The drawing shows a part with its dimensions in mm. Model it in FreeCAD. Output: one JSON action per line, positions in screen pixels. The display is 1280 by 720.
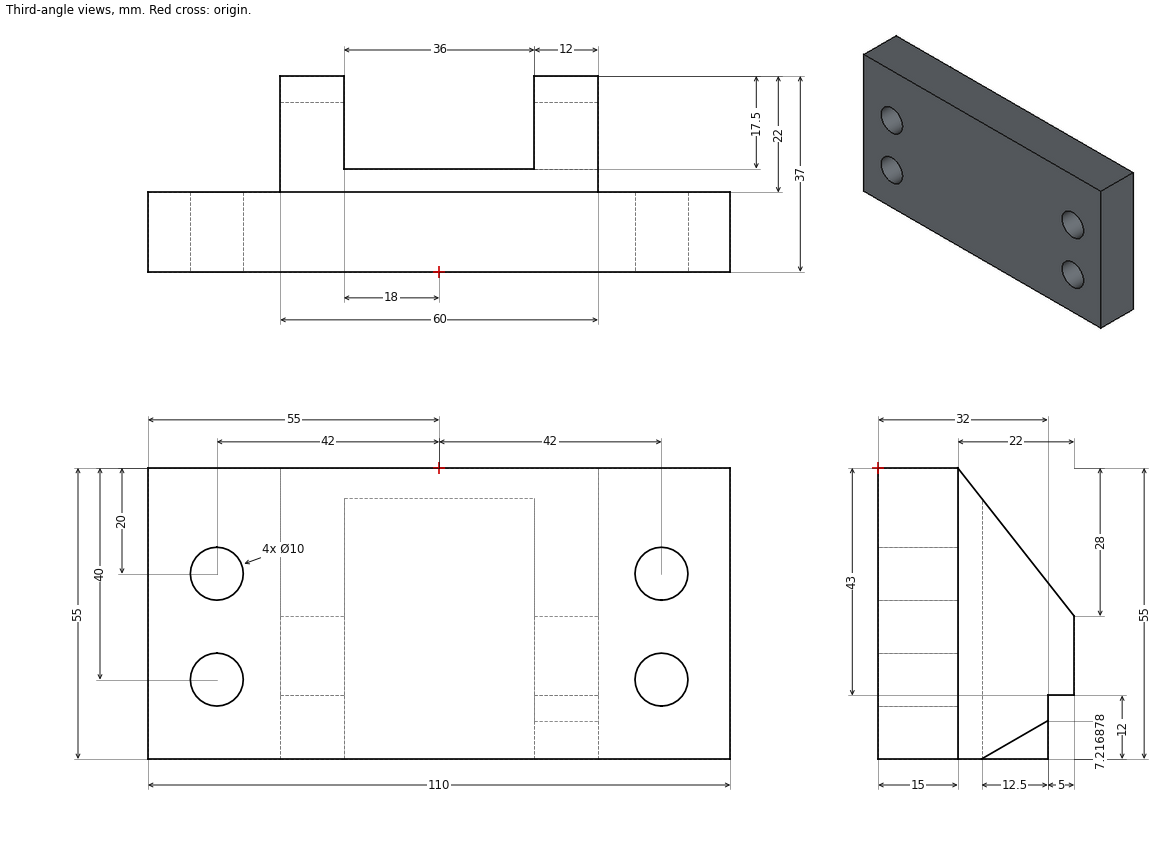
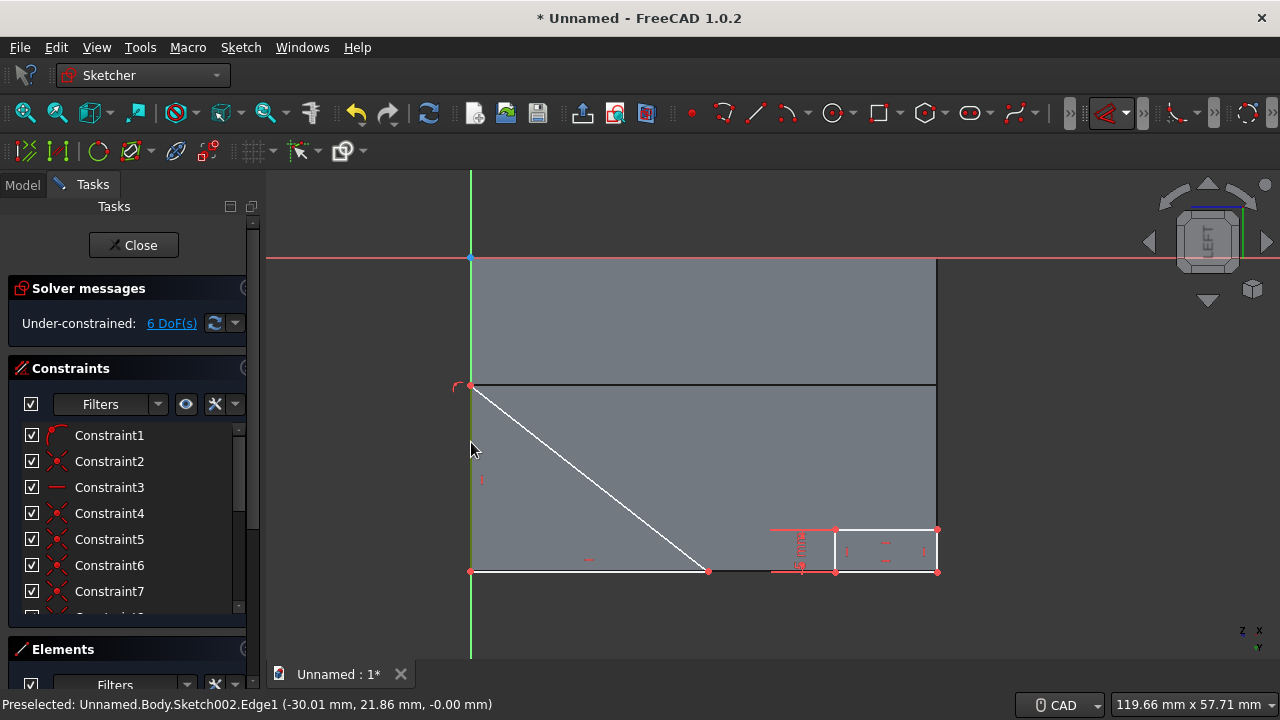
{"action": "left_click", "coordinate": [1128, 114]}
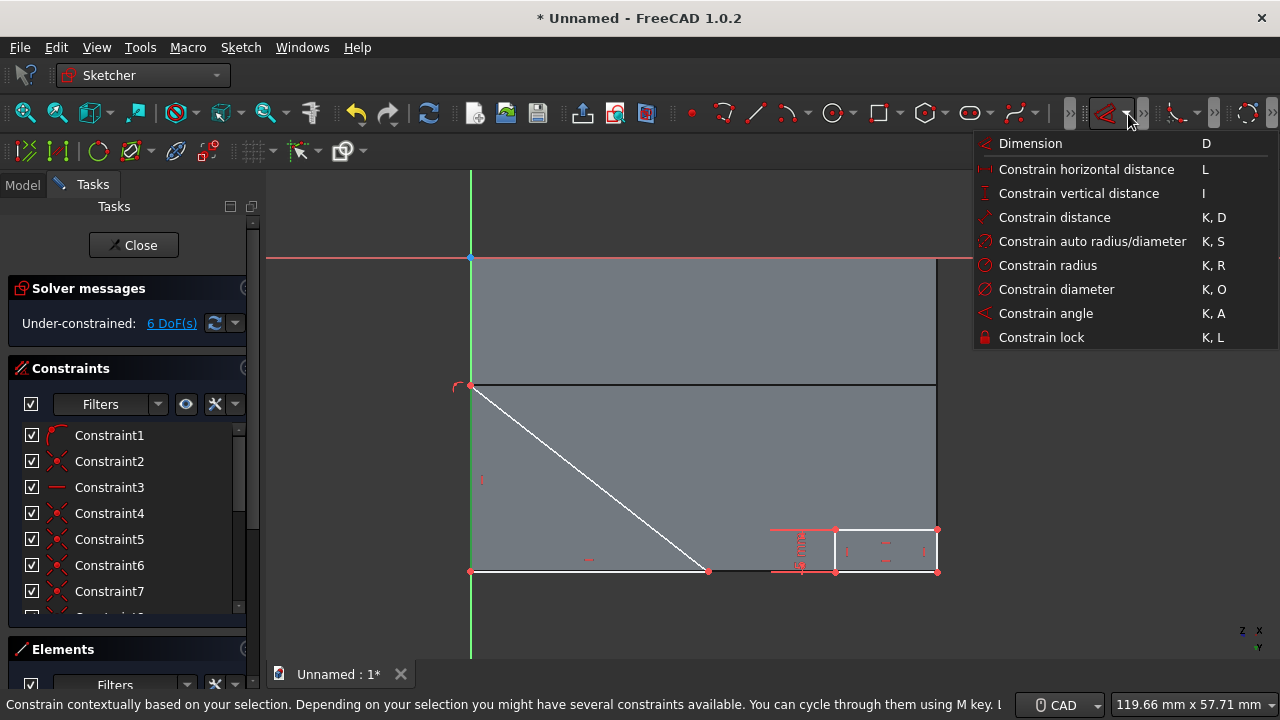
{"action": "left_click", "coordinate": [1126, 193]}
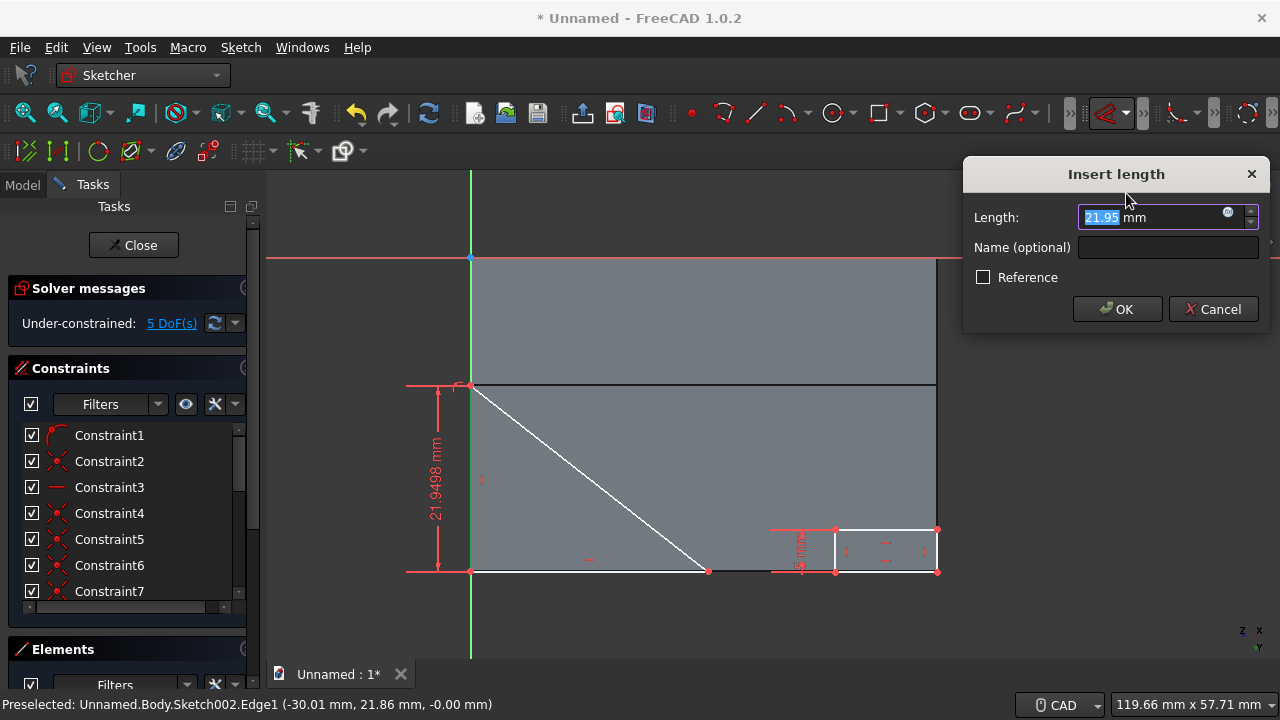
{"action": "type", "text": "22"}
{"action": "key", "text": "Return"}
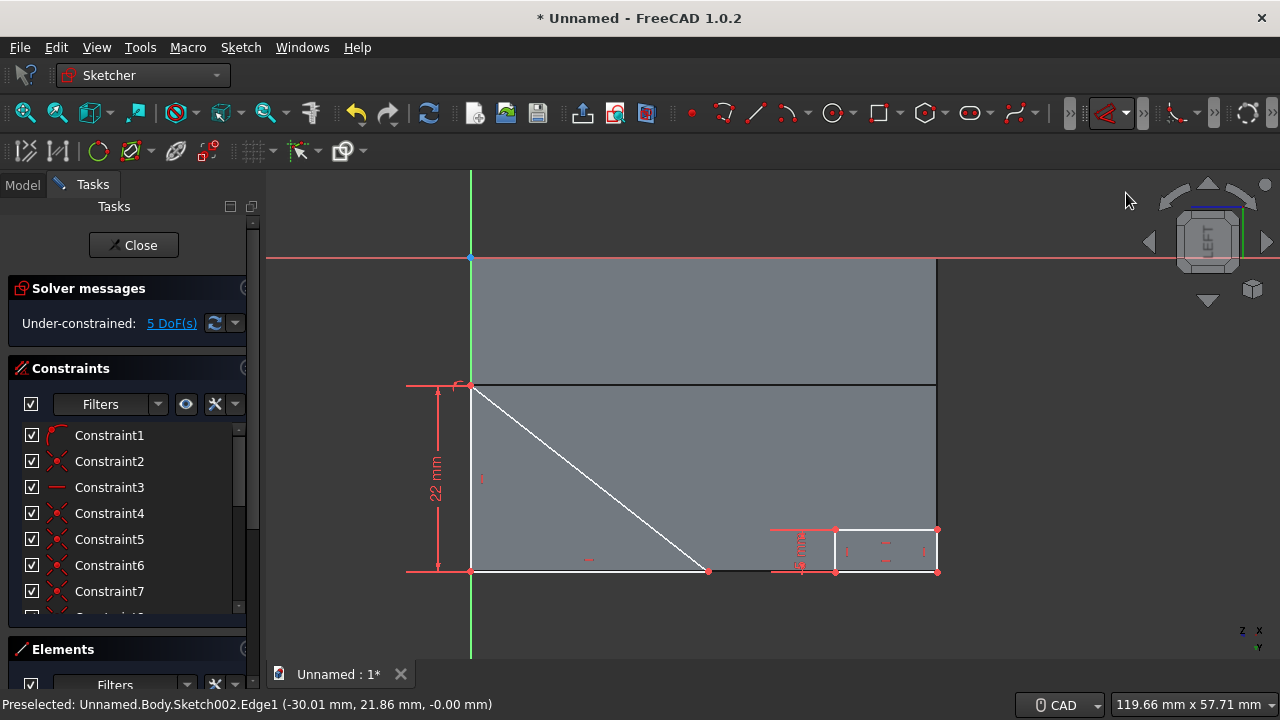
{"action": "left_click", "coordinate": [542, 572]}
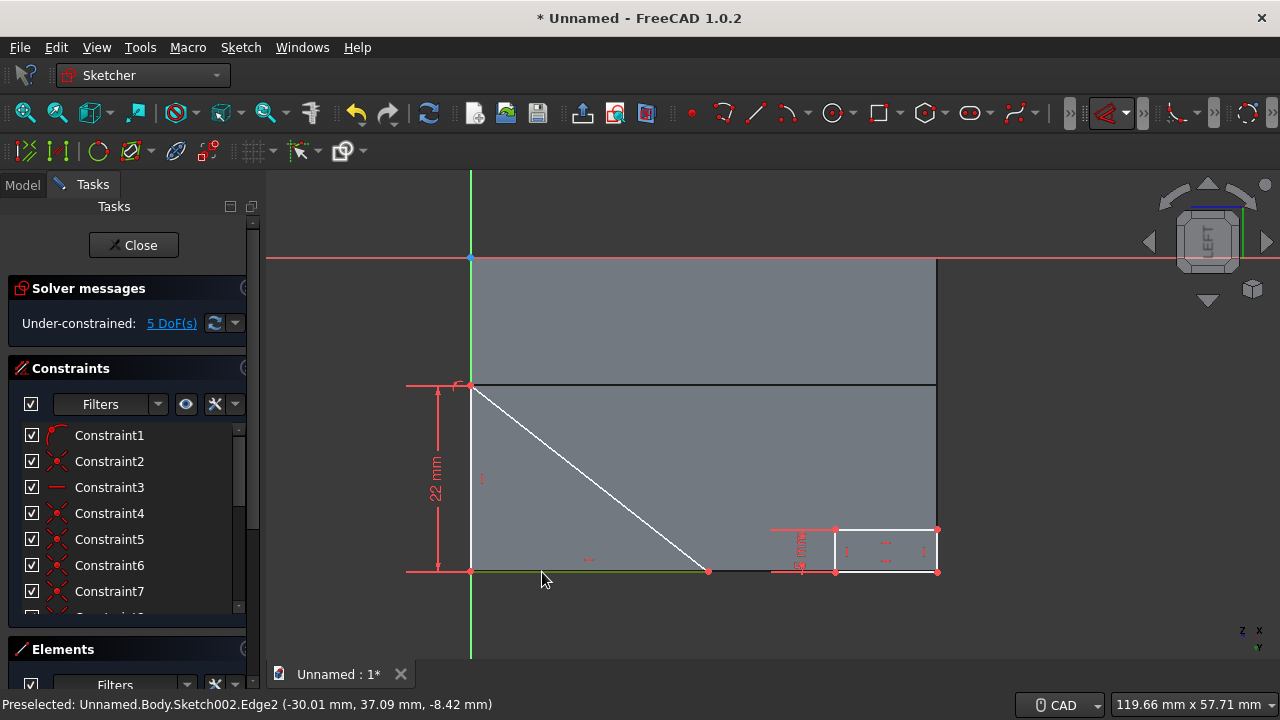
{"action": "left_click", "coordinate": [1128, 114]}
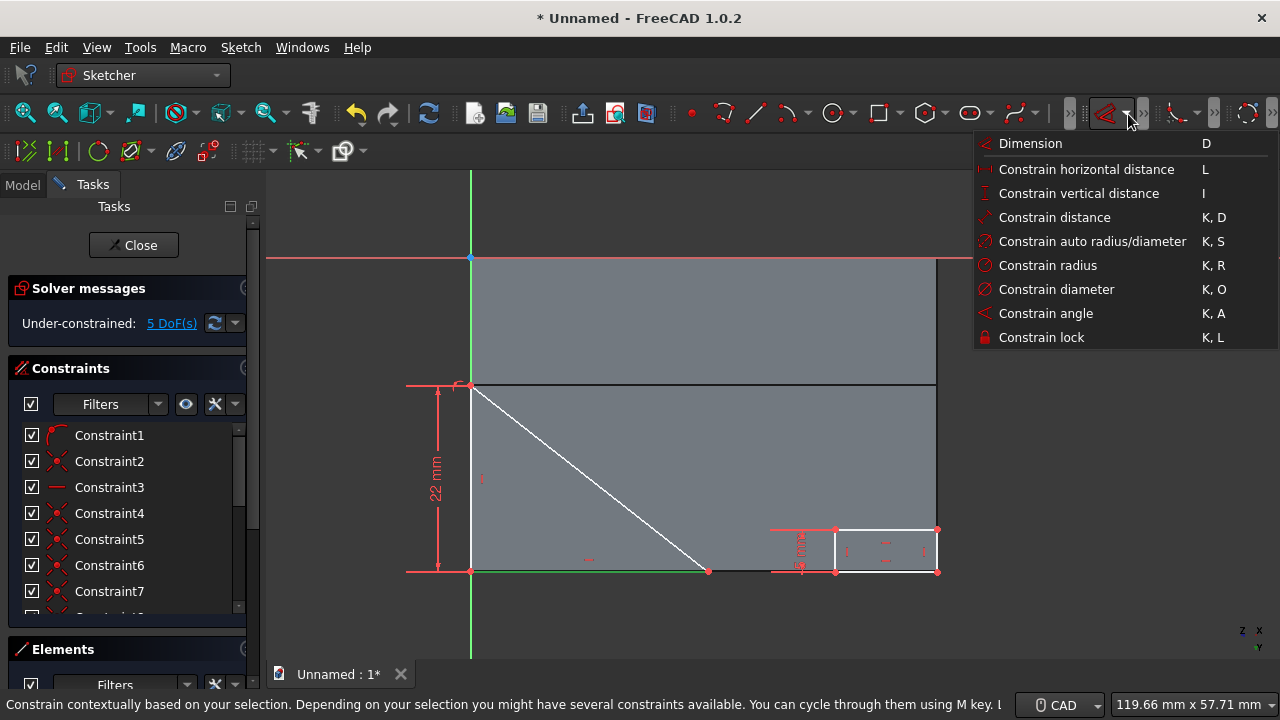
{"action": "left_click", "coordinate": [1126, 169]}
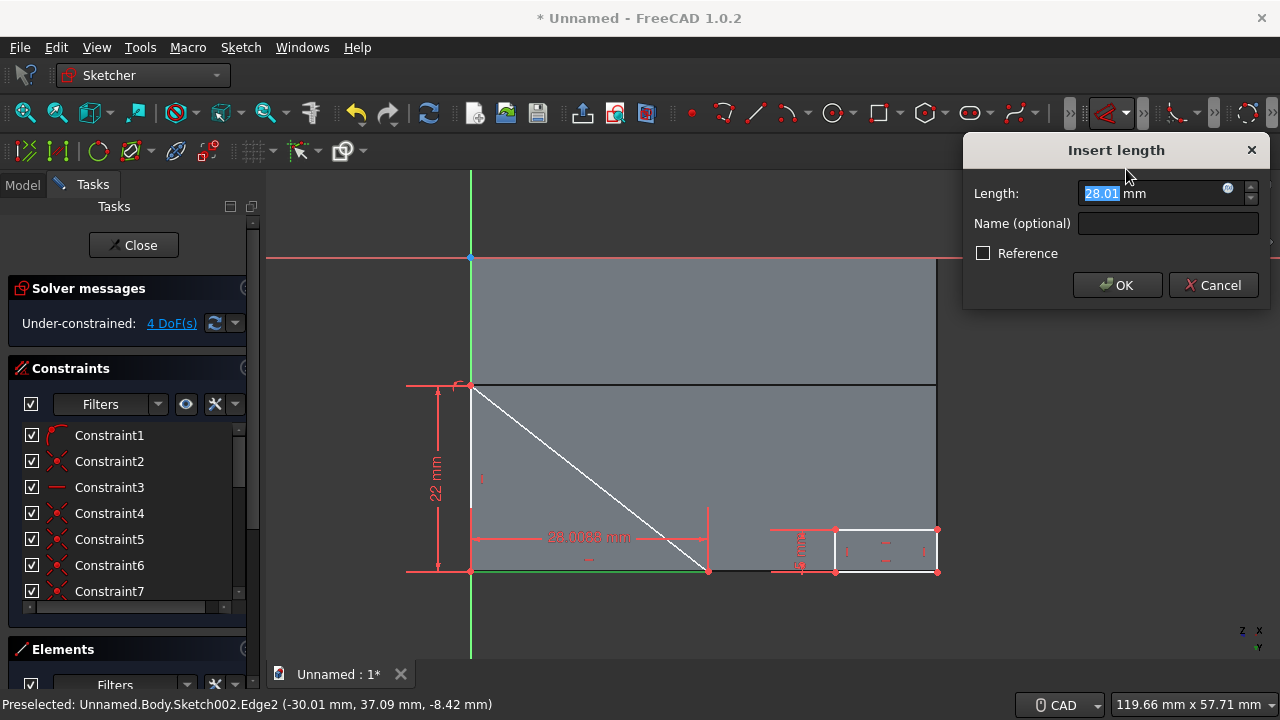
{"action": "type", "text": "28"}
{"action": "key", "text": "Return"}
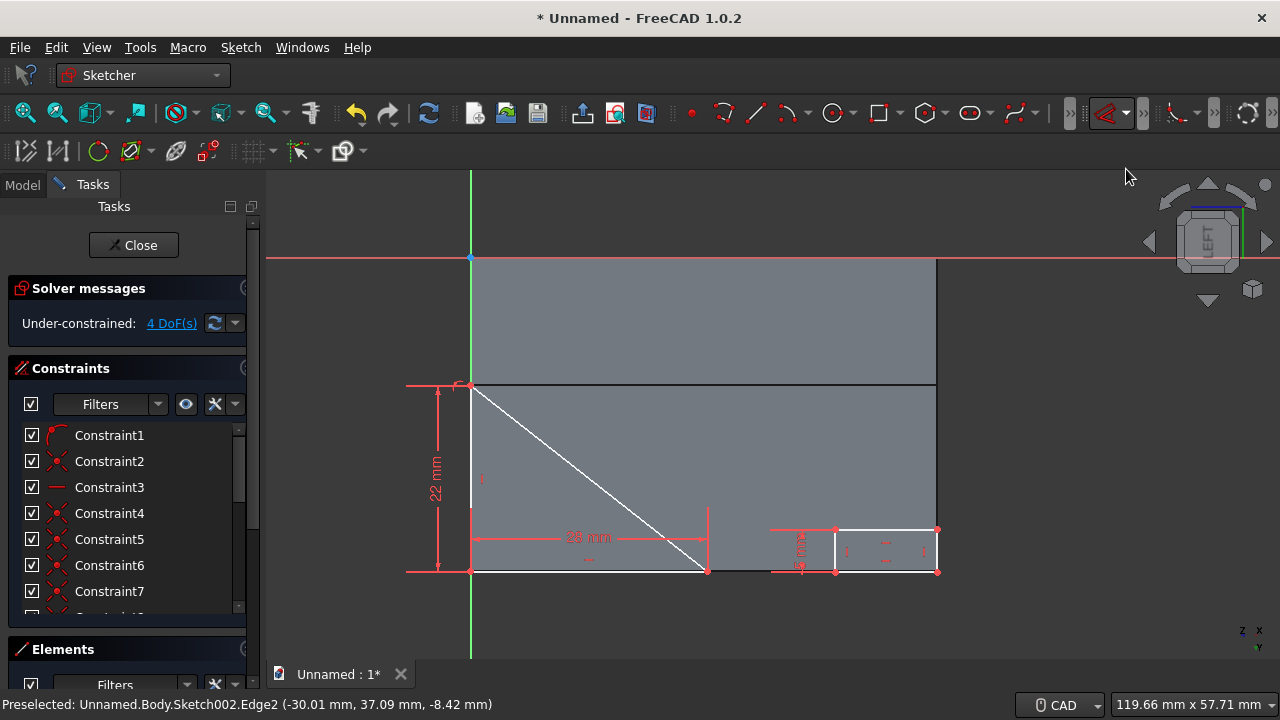
{"action": "left_click", "coordinate": [866, 572]}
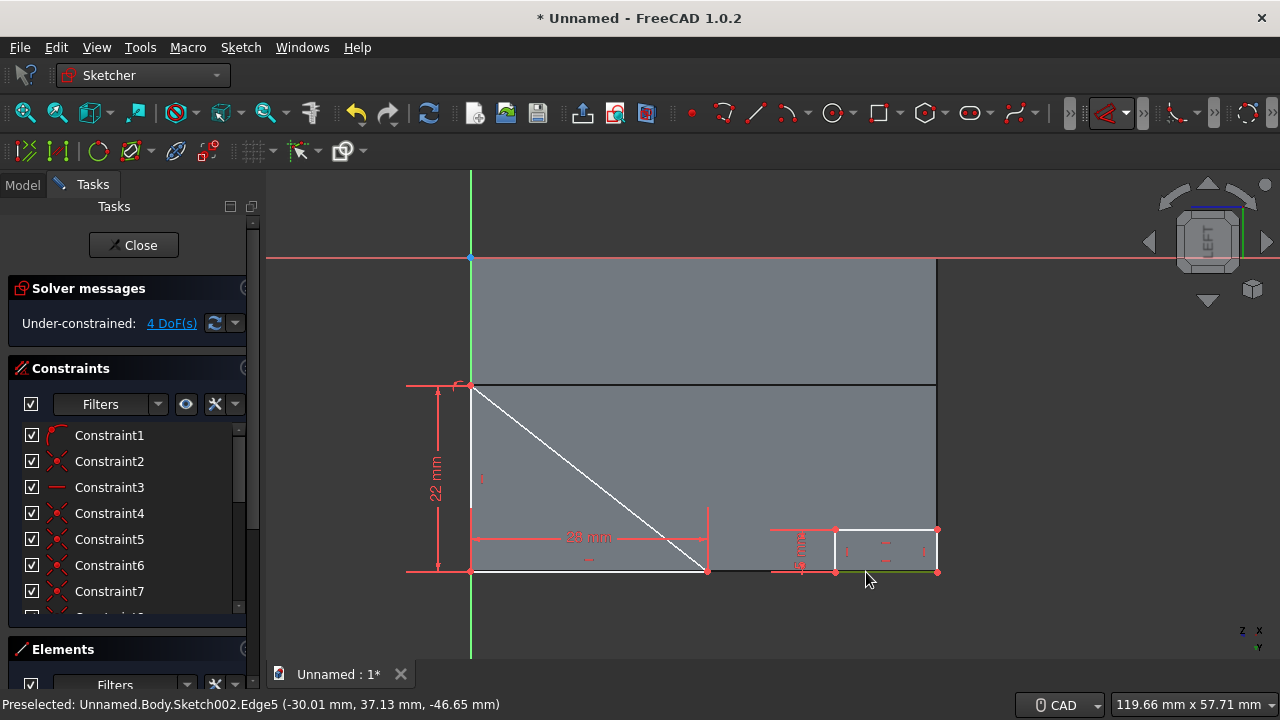
{"action": "left_click", "coordinate": [1128, 114]}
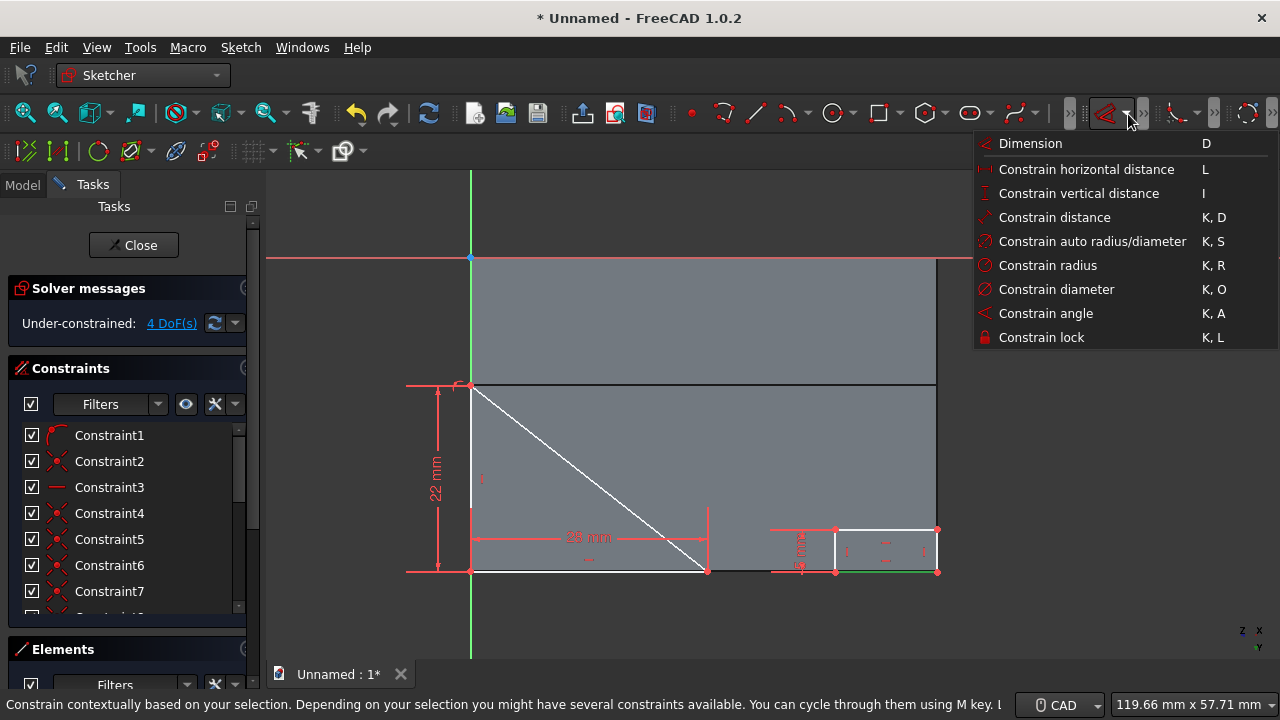
{"action": "left_click", "coordinate": [1126, 169]}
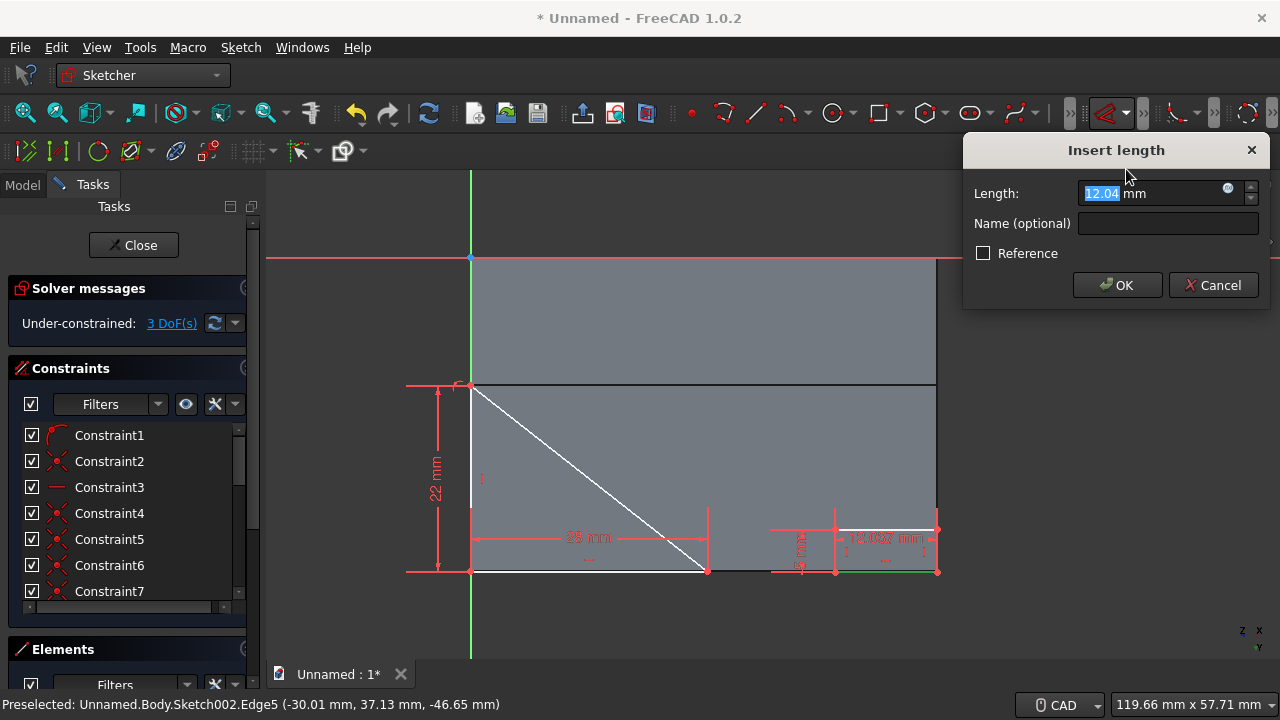
{"action": "type", "text": "12"}
{"action": "key", "text": "Return"}